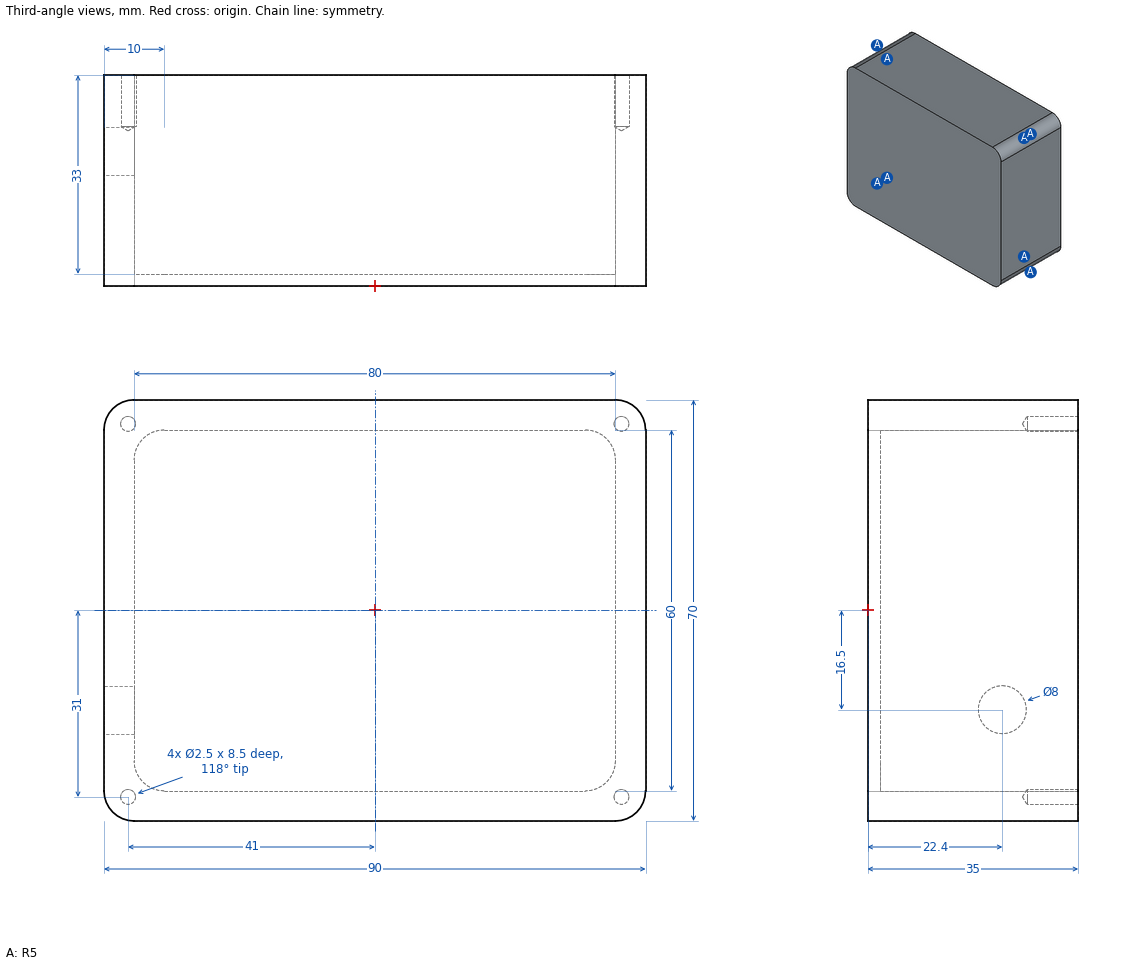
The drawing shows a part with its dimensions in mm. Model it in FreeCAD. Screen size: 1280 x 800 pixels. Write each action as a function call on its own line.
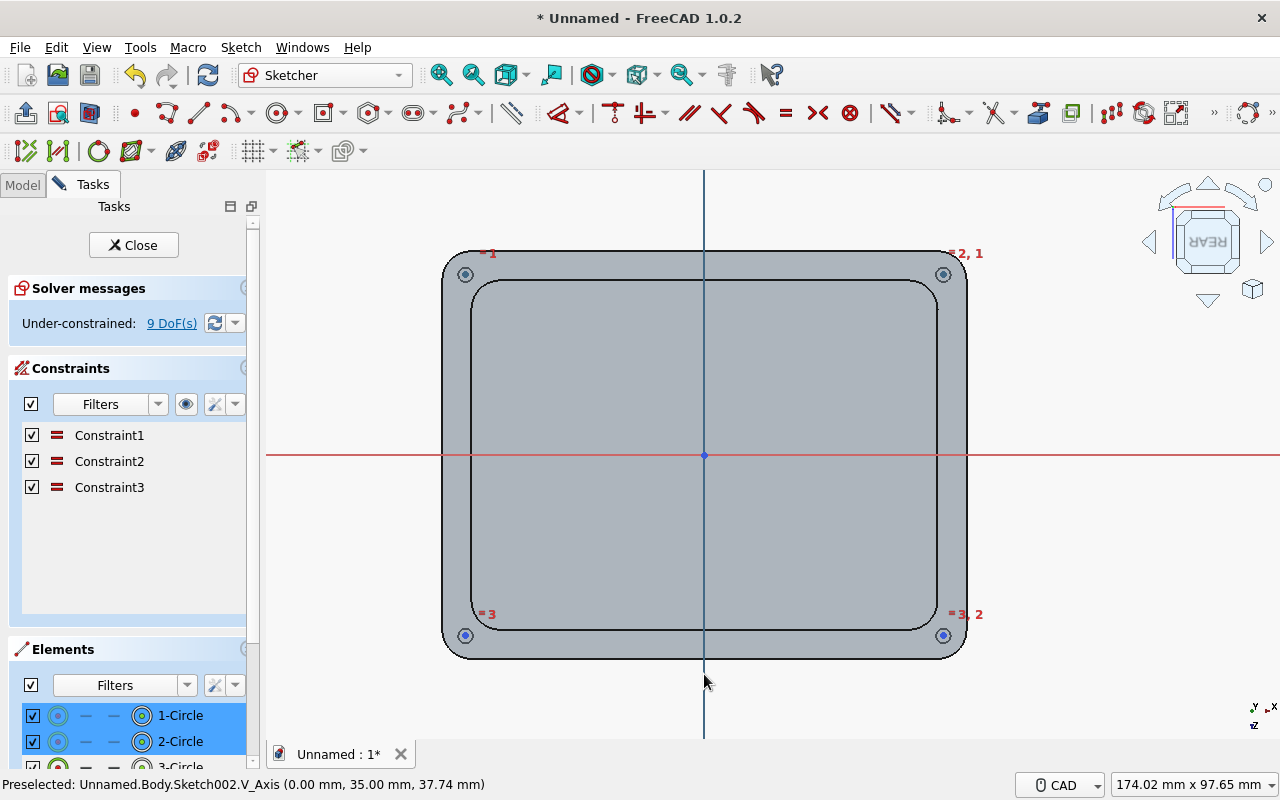
click(818, 114)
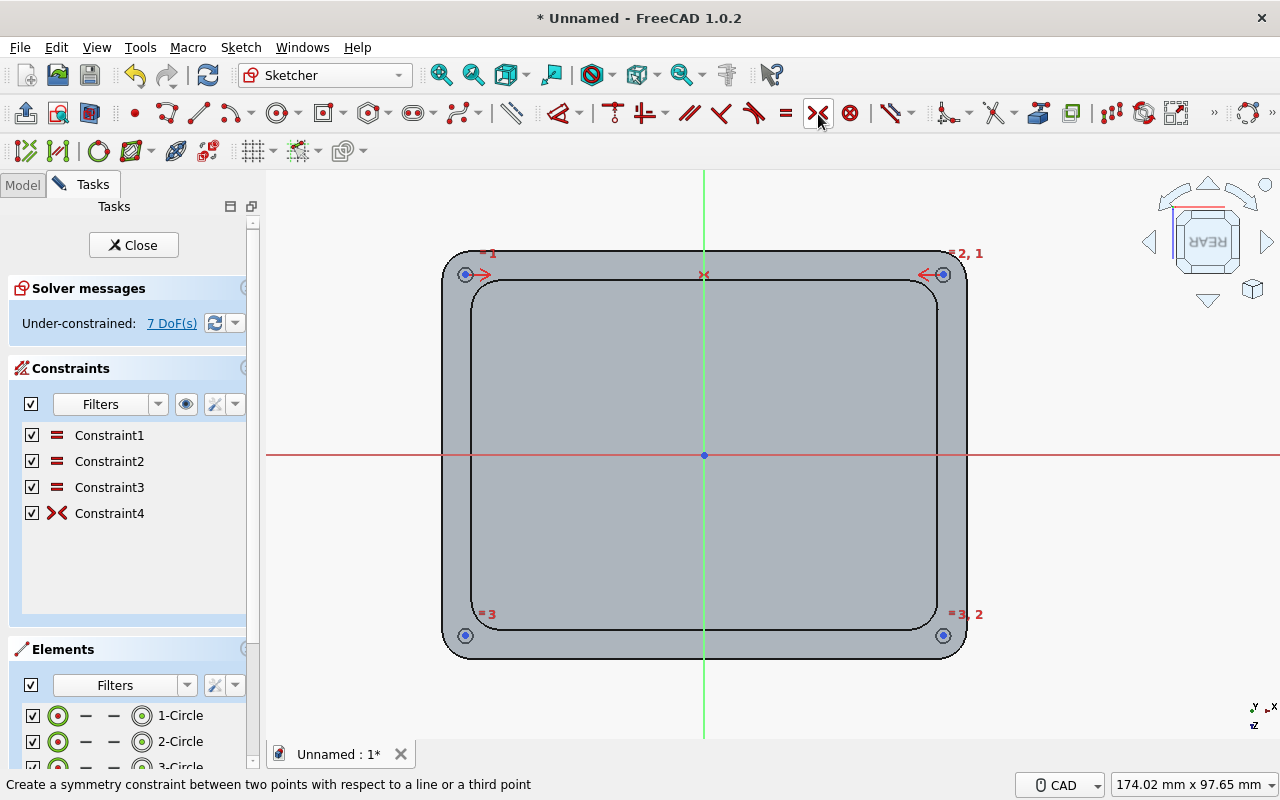
click(943, 275)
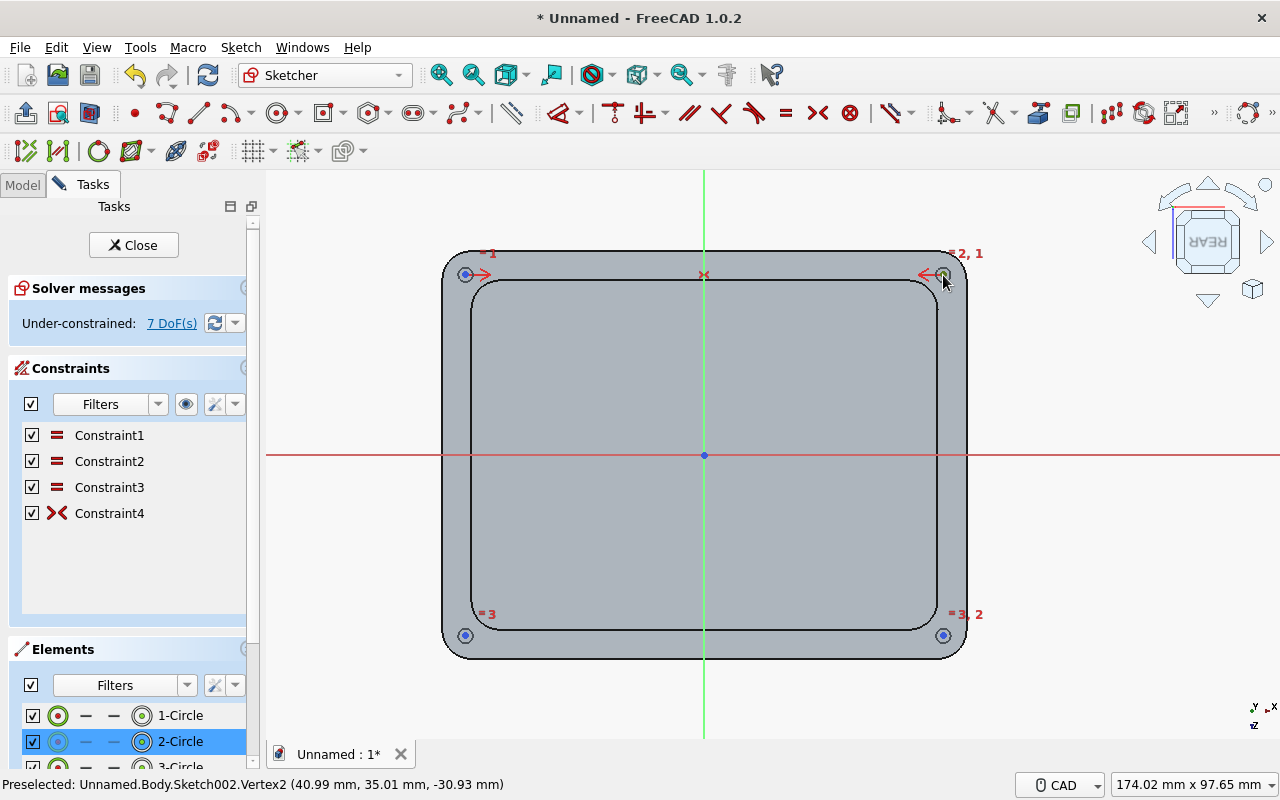
click(943, 636)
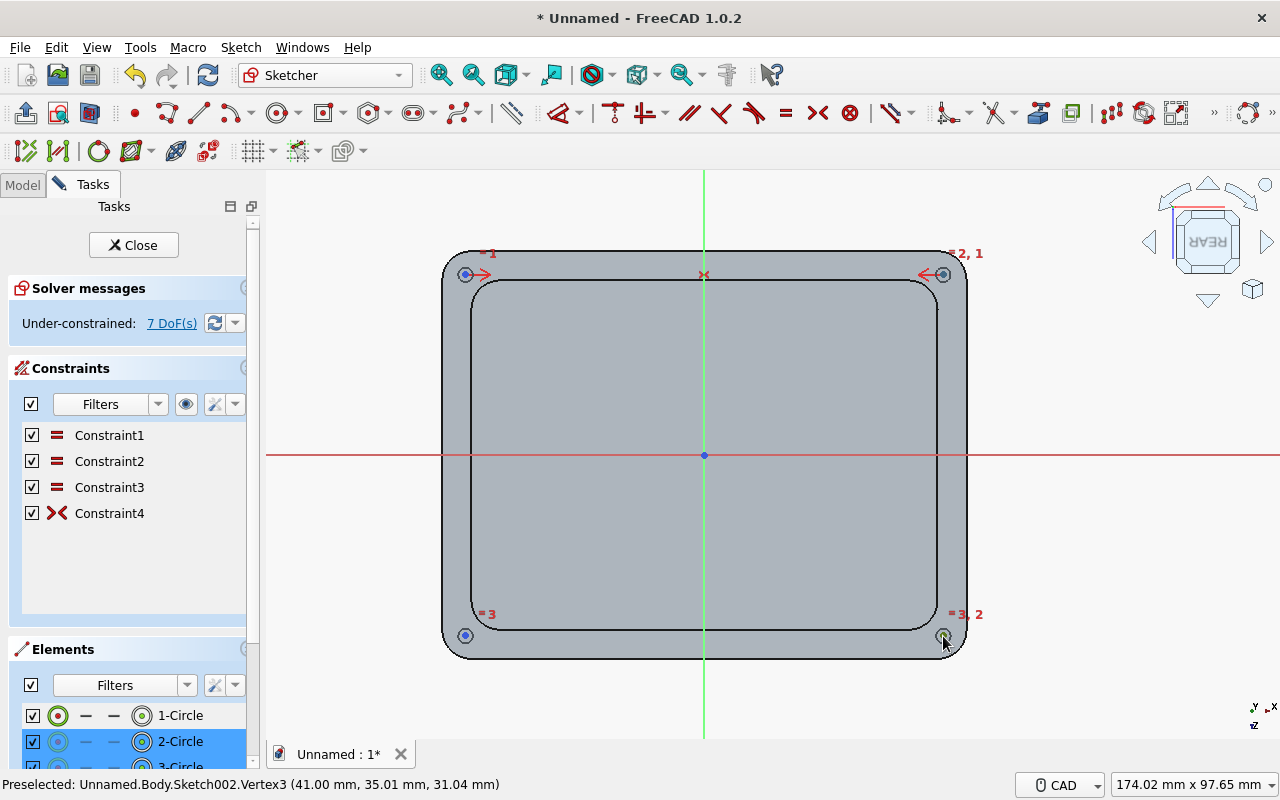
click(353, 455)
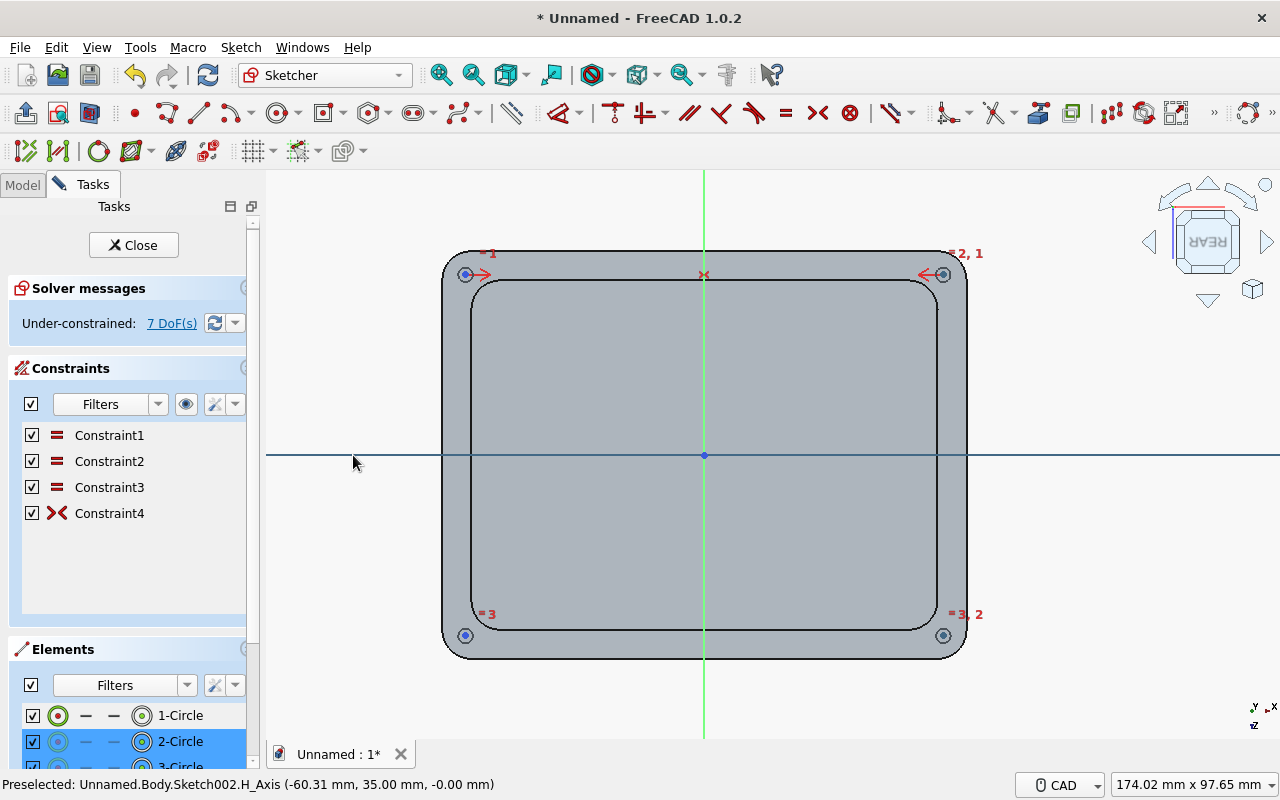
click(818, 114)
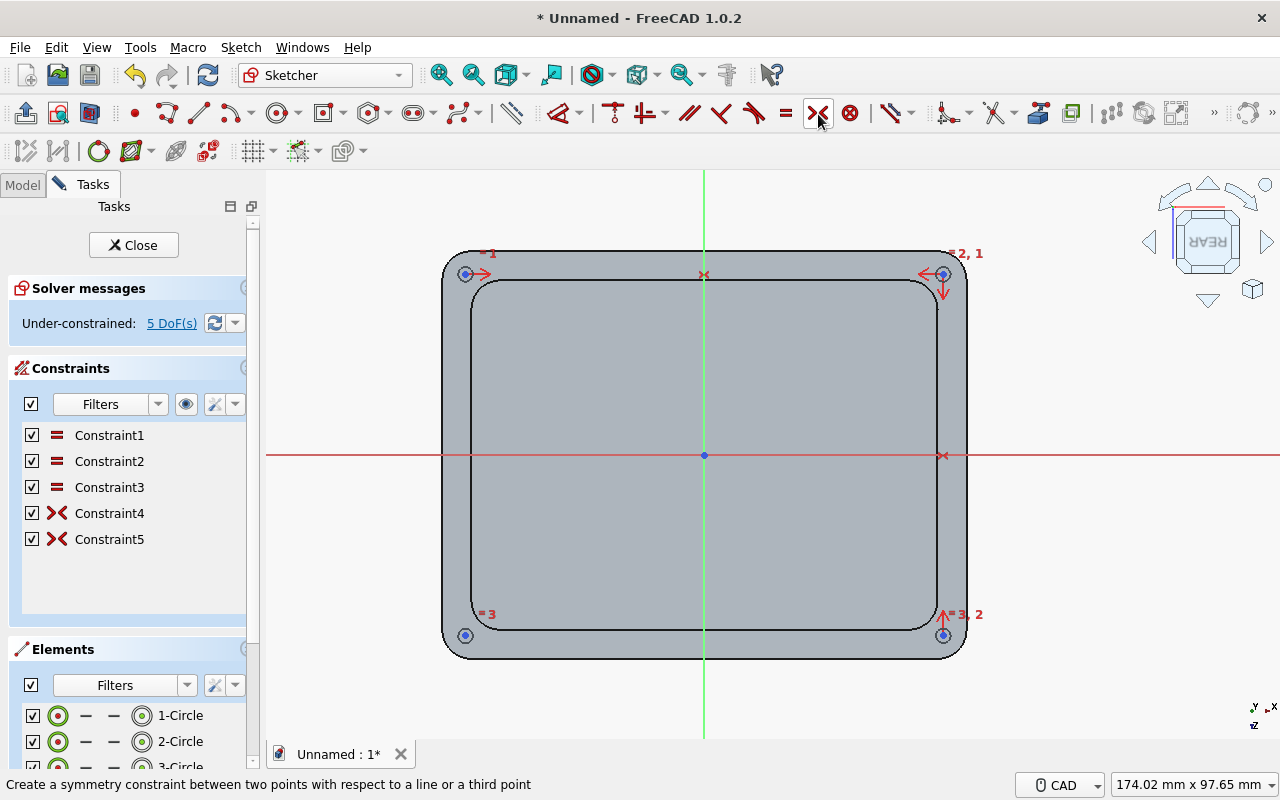
click(466, 274)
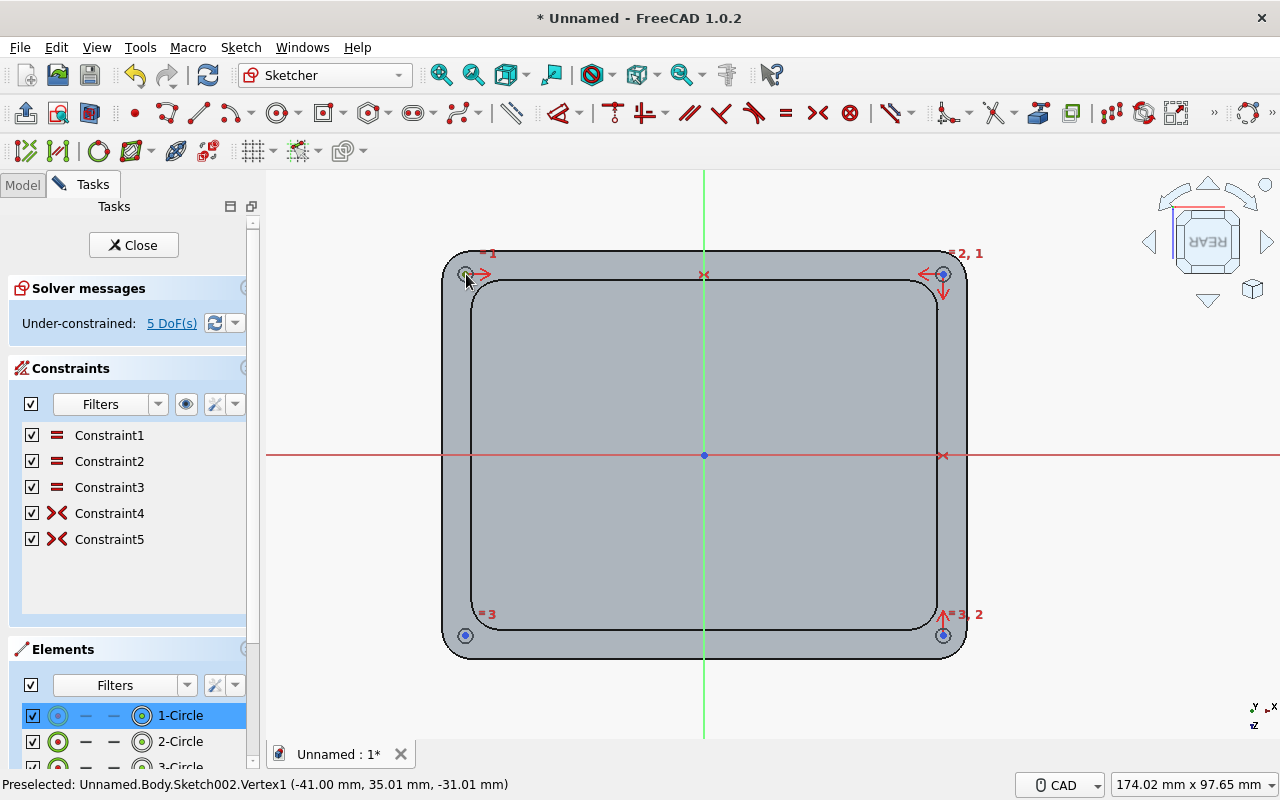
click(466, 636)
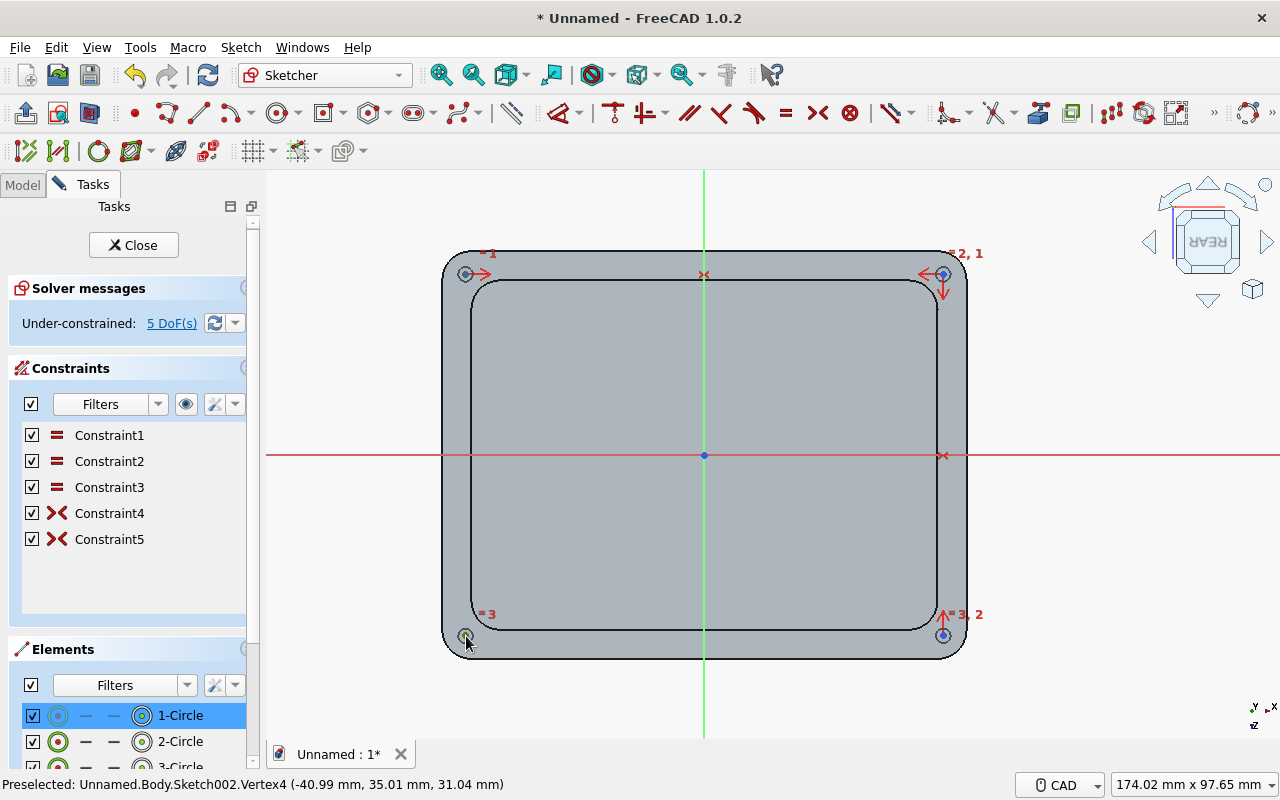
click(353, 455)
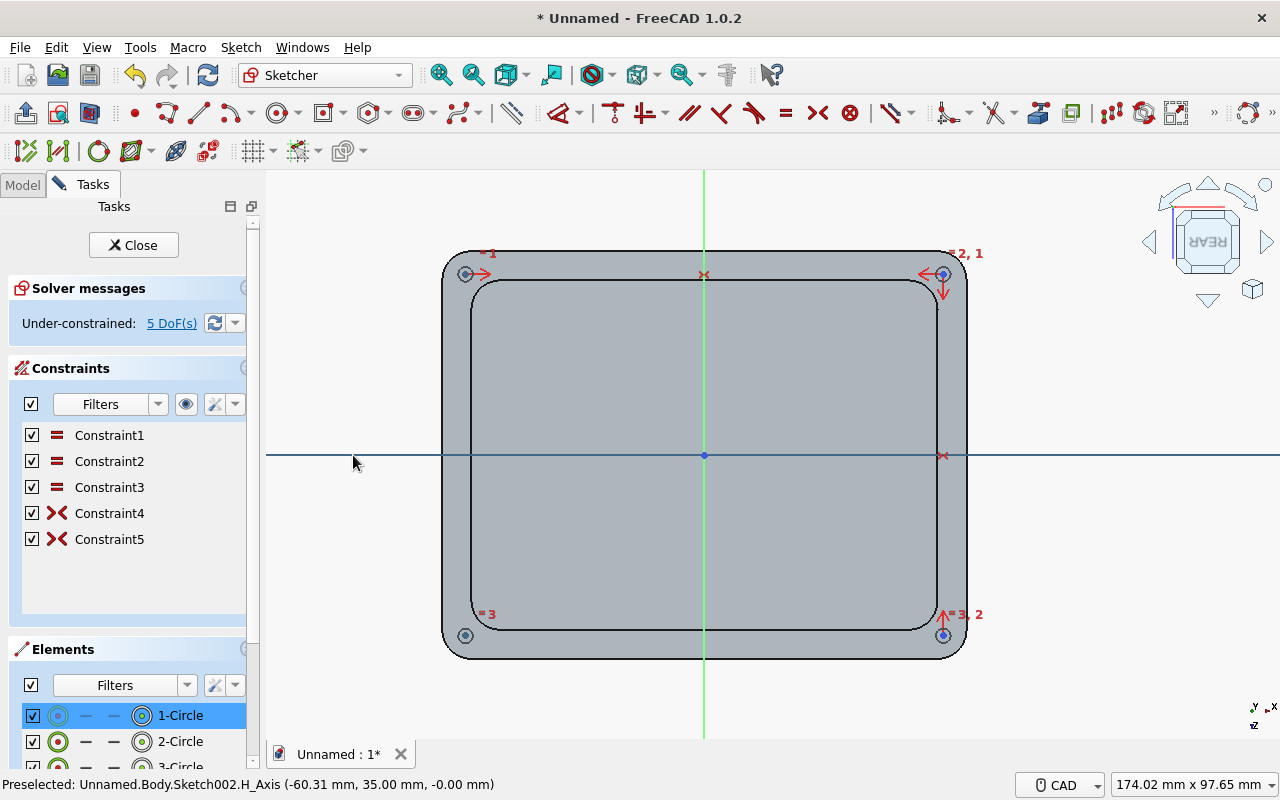
click(818, 114)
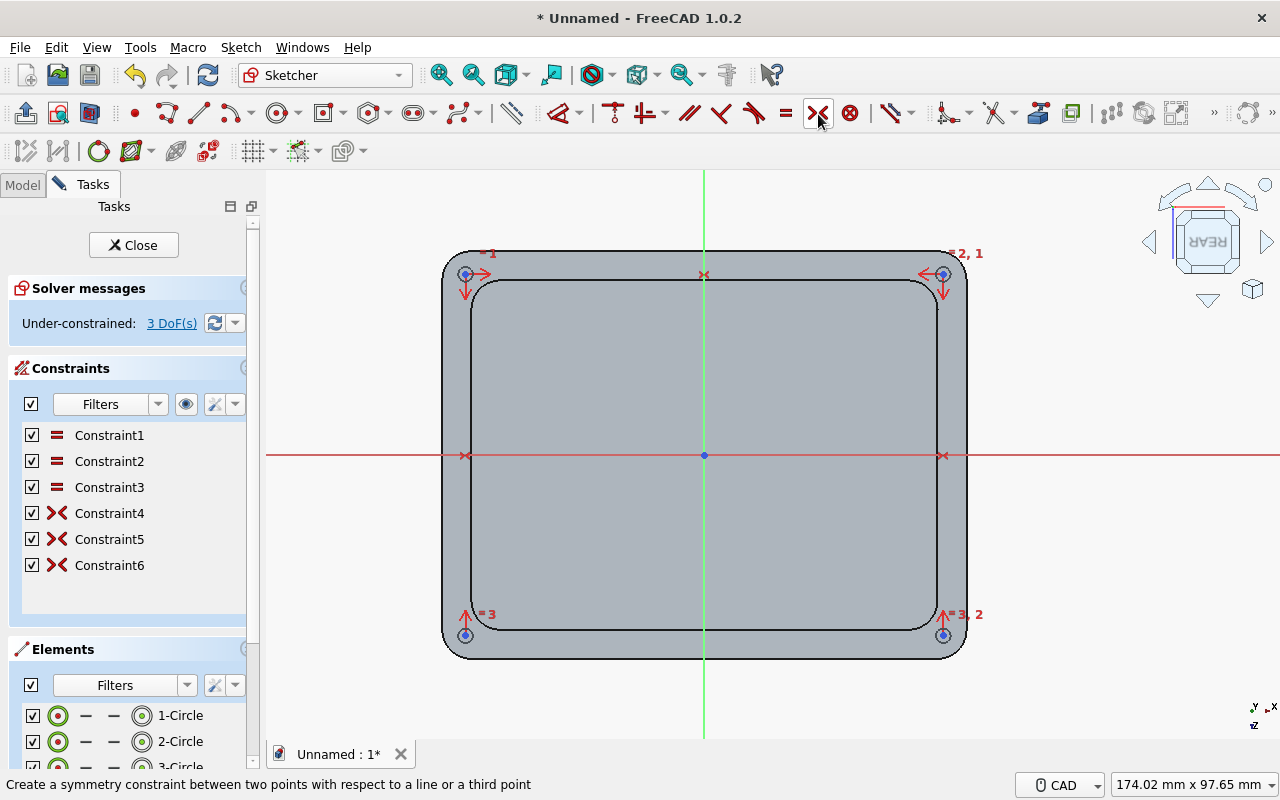
key(d)